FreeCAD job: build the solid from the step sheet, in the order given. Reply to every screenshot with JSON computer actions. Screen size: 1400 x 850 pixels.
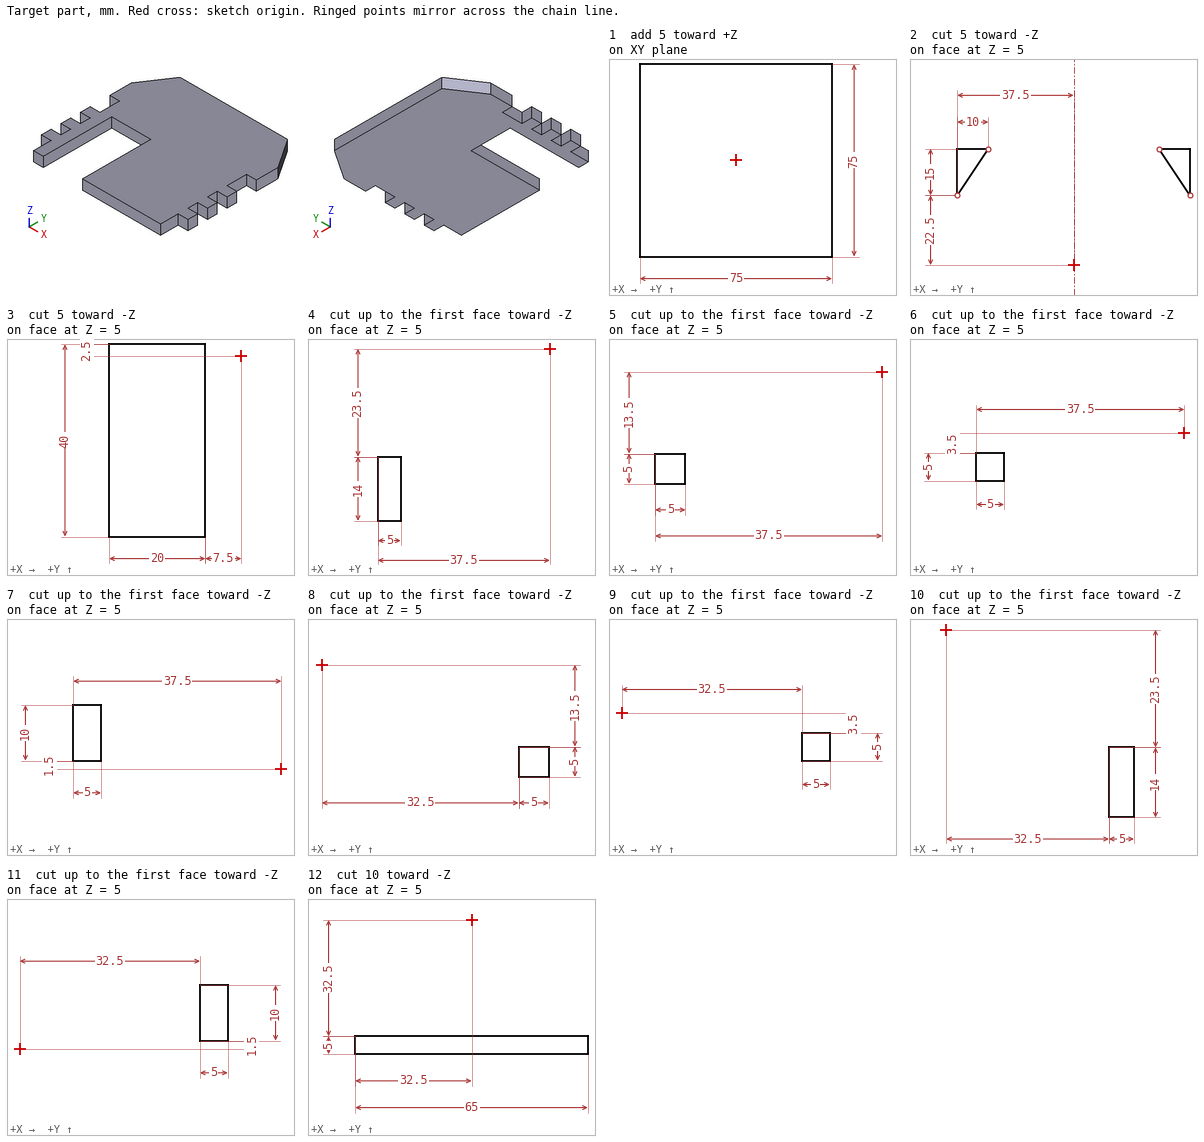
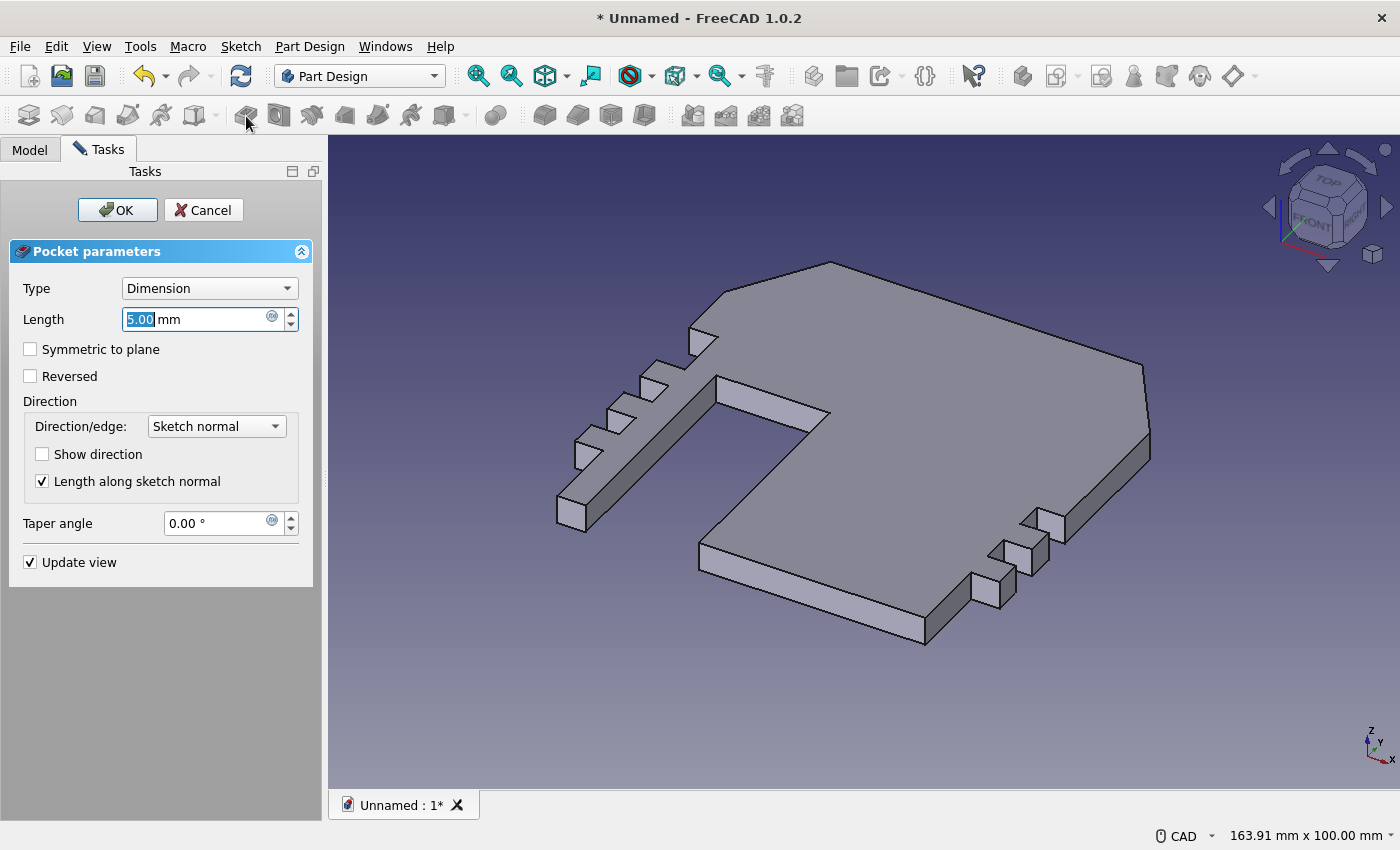
{"action": "left_click", "coordinate": [210, 288]}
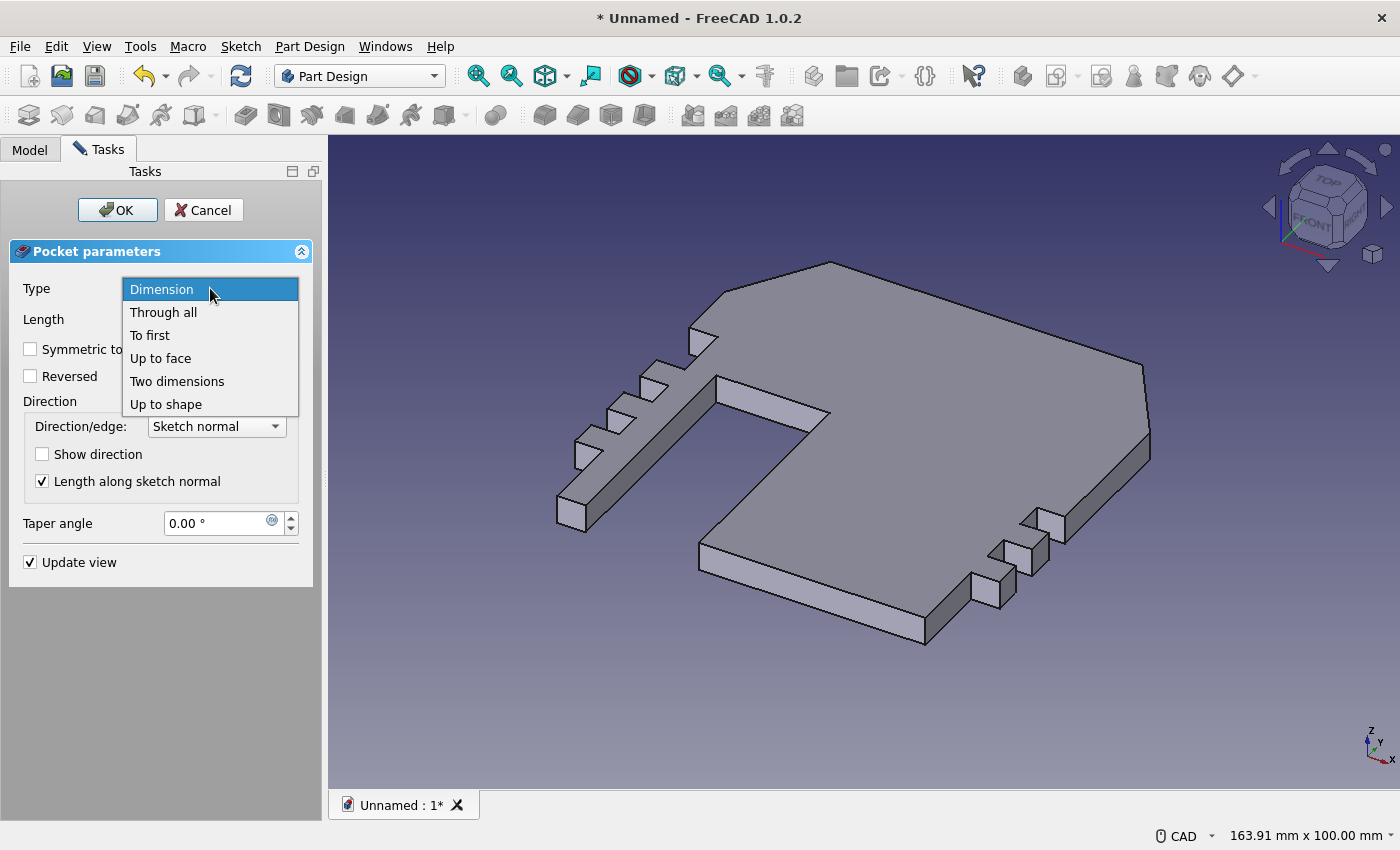
{"action": "left_click", "coordinate": [208, 336]}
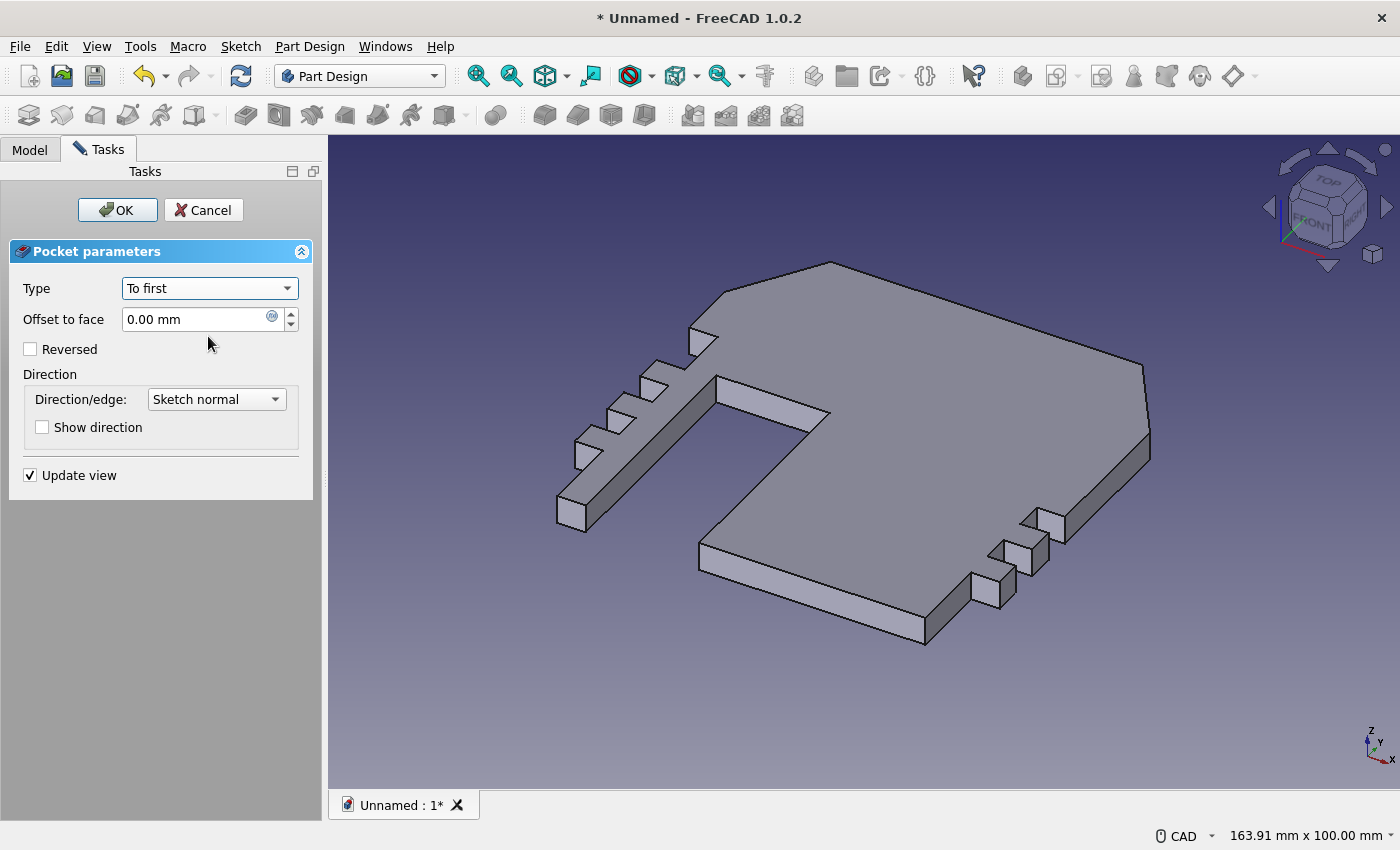
{"action": "left_click", "coordinate": [118, 210]}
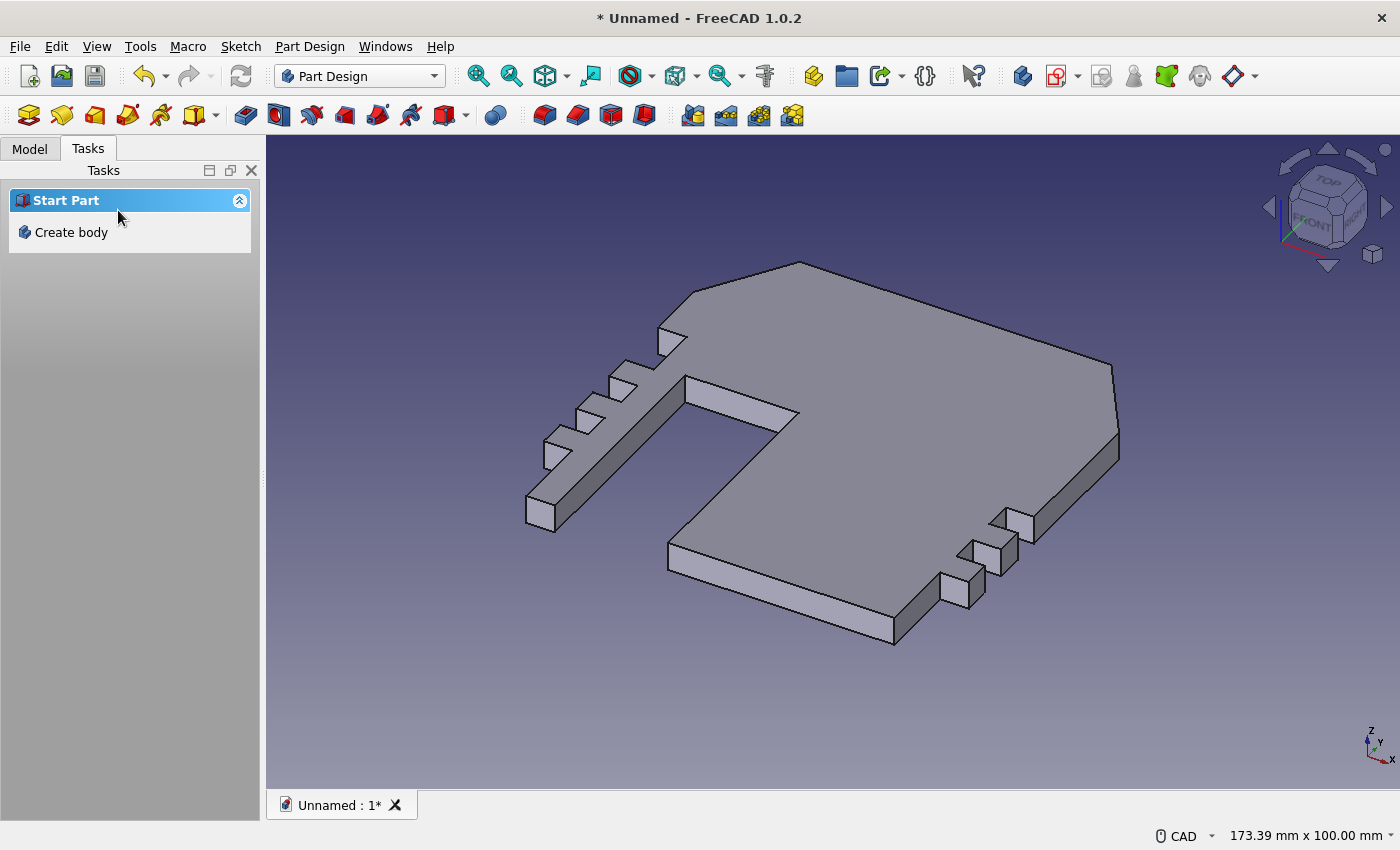
{"action": "left_click", "coordinate": [929, 420]}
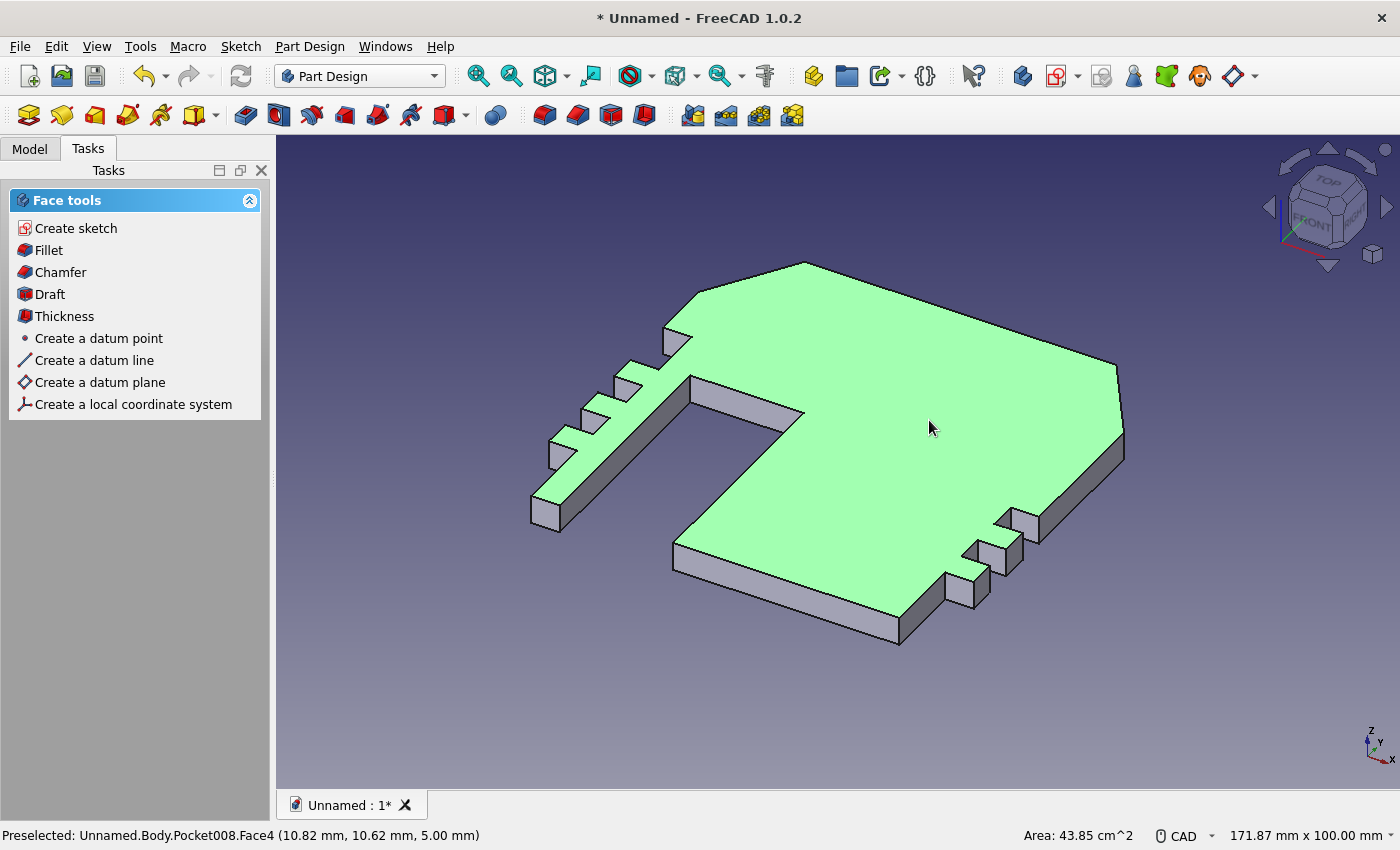
{"action": "left_click", "coordinate": [1056, 76]}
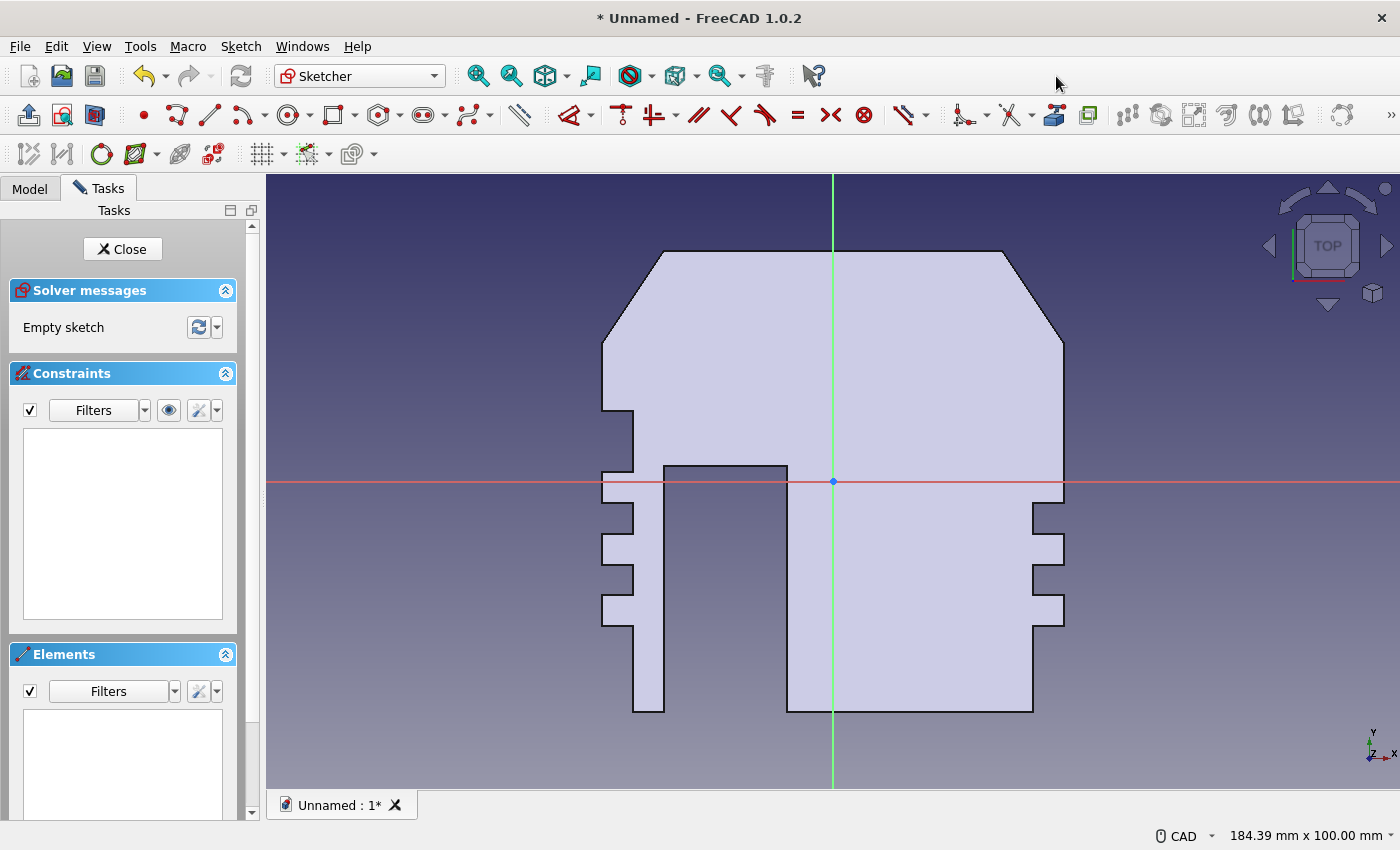
{"action": "scroll", "coordinate": [1104, 434], "scroll_direction": "up", "scroll_amount": 9}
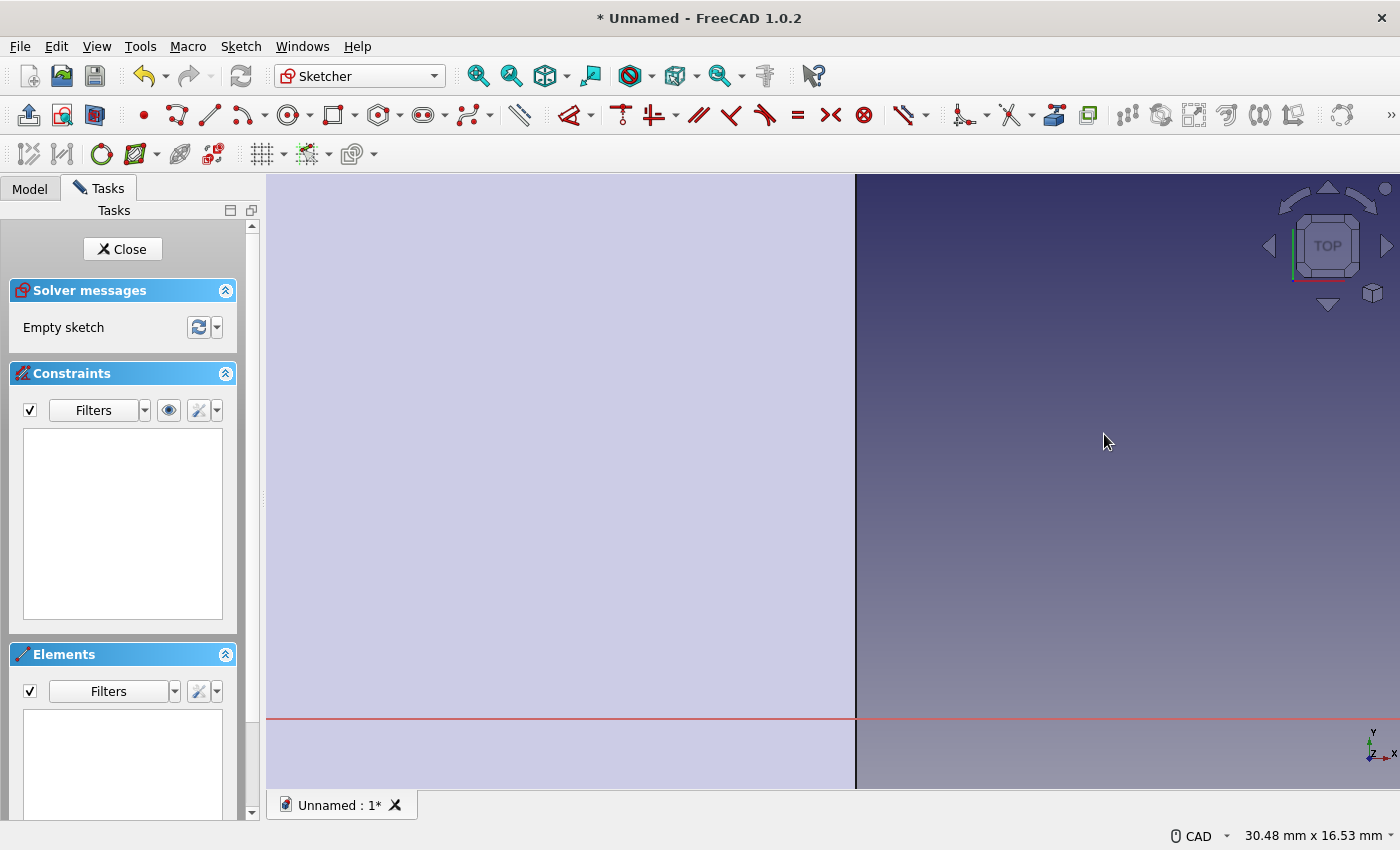
{"action": "left_click", "coordinate": [332, 116]}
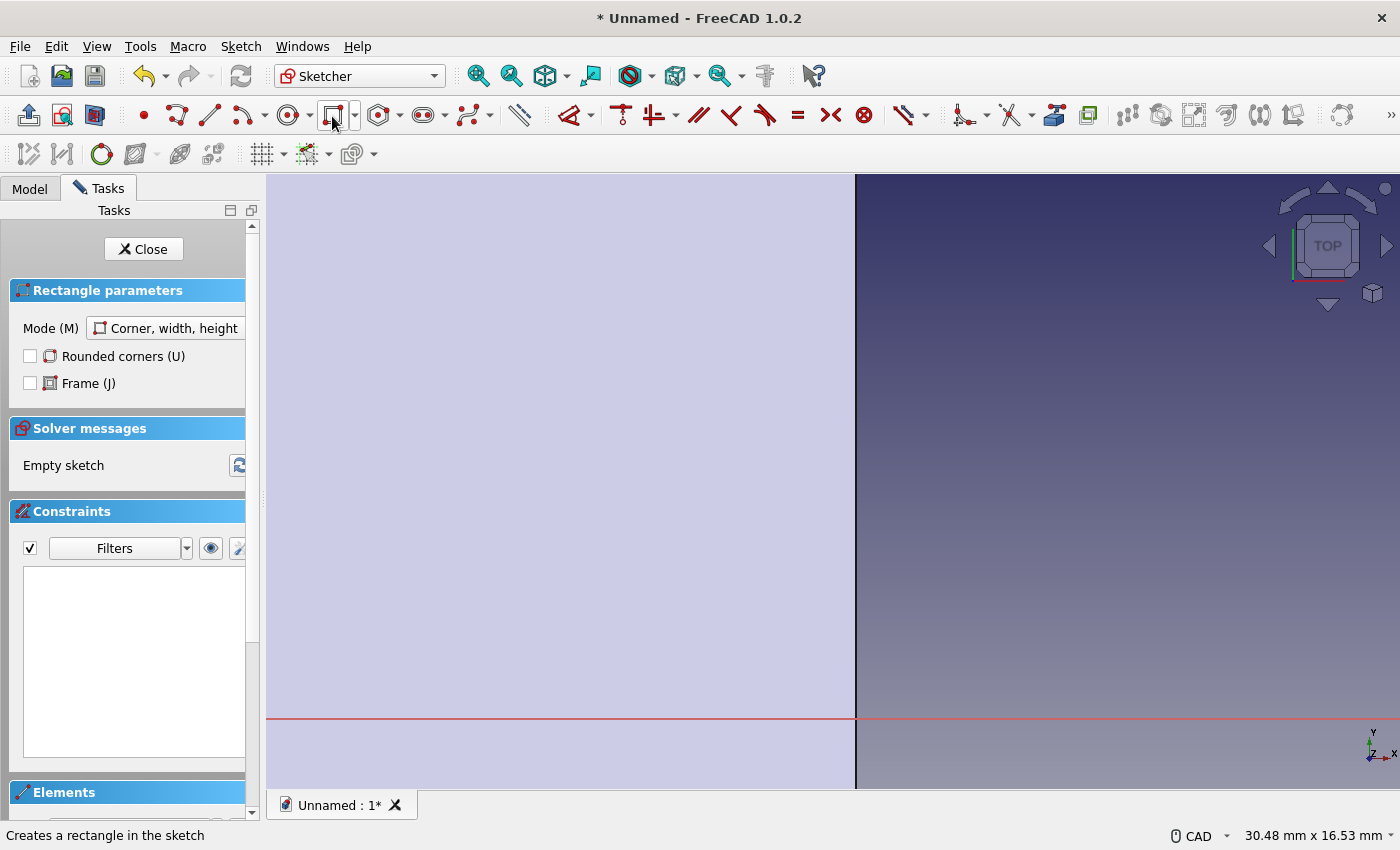
{"action": "left_click", "coordinate": [670, 291]}
{"action": "left_click", "coordinate": [856, 663]}
{"action": "key", "text": "Escape"}